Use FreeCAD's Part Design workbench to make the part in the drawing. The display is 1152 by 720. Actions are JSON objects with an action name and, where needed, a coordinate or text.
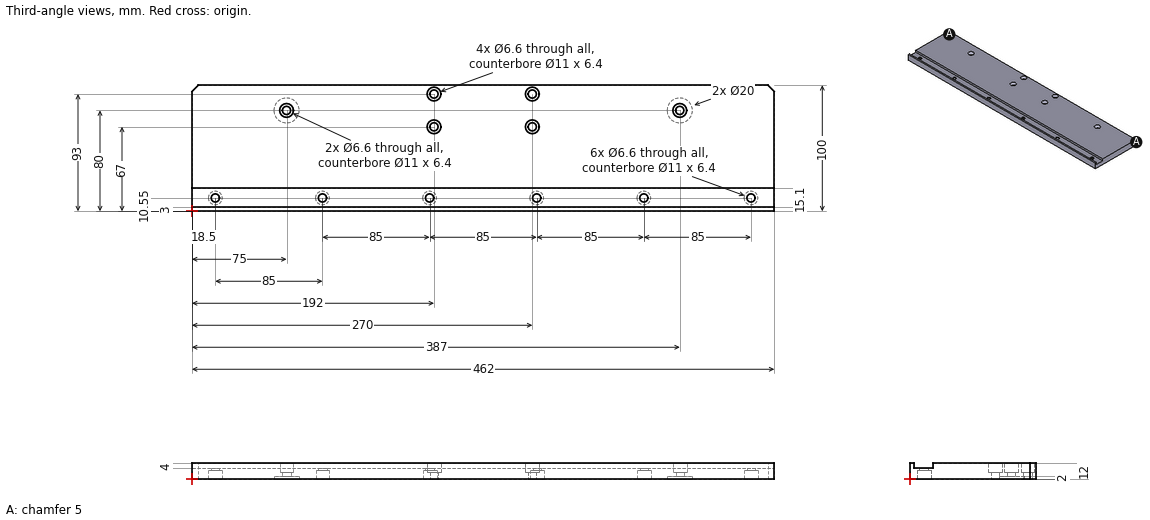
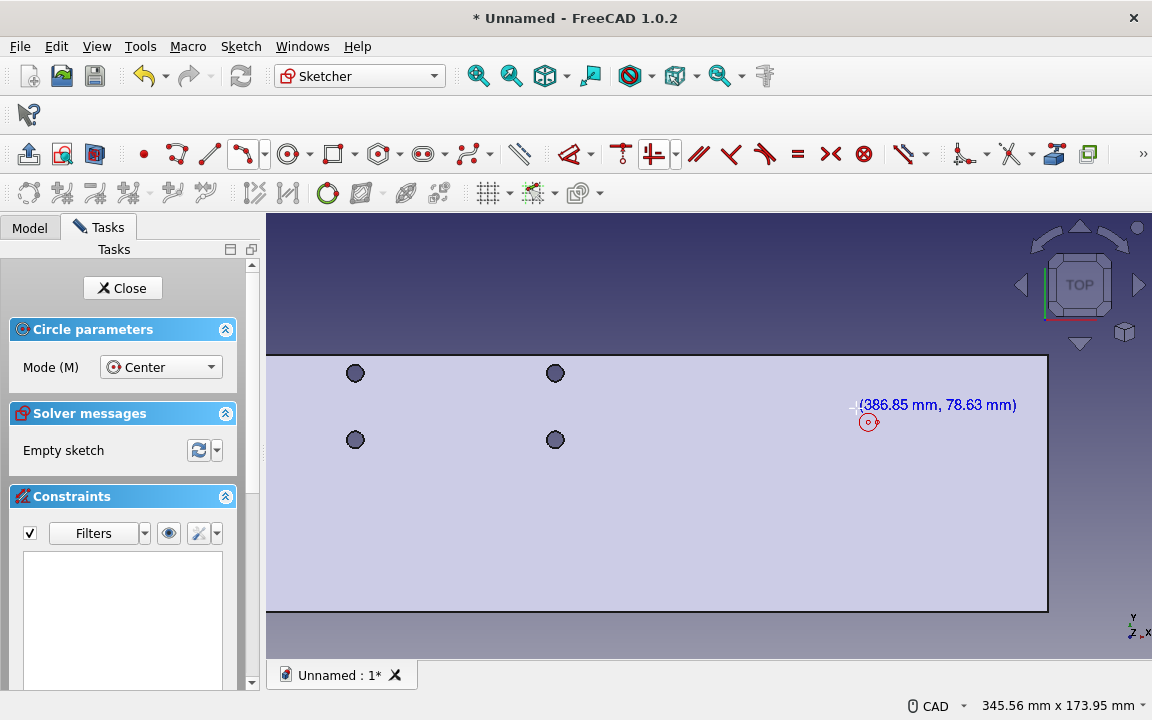
{"action": "left_click", "coordinate": [855, 406]}
{"action": "mouse_move", "coordinate": [873, 388]}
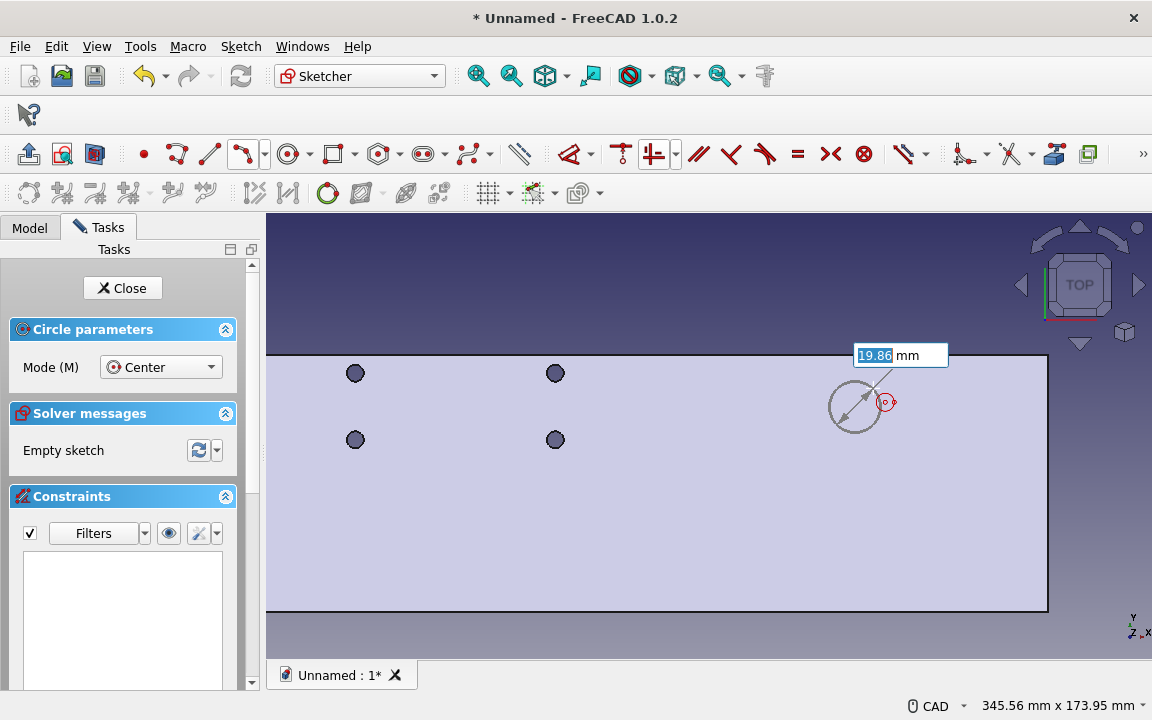
{"action": "type", "text": "20"}
{"action": "key", "text": "Return"}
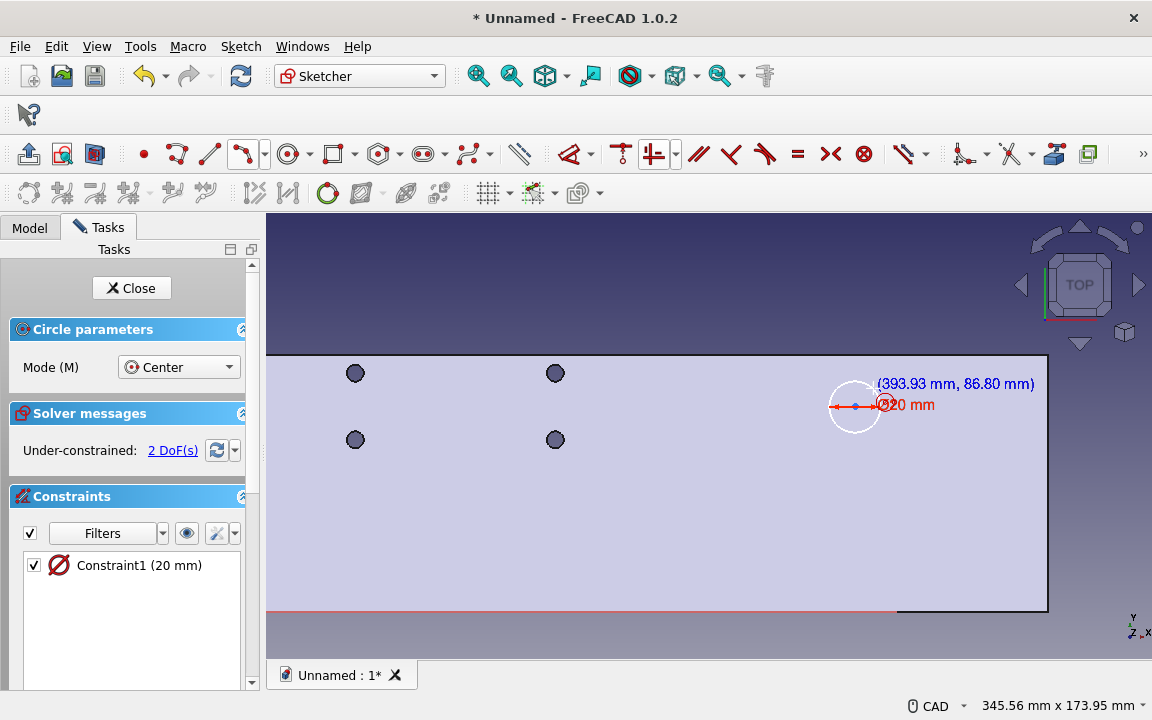
{"action": "scroll", "coordinate": [860, 387], "scroll_direction": "down", "scroll_amount": 4}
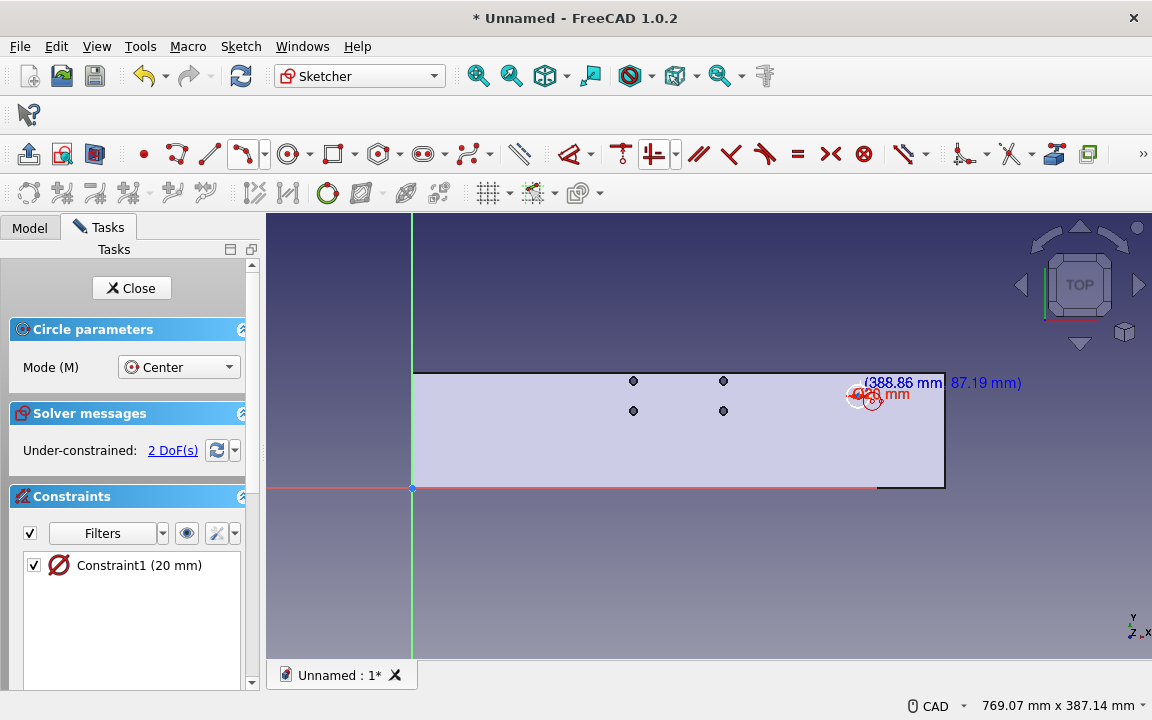
{"action": "scroll", "coordinate": [499, 396], "scroll_direction": "up", "scroll_amount": 4}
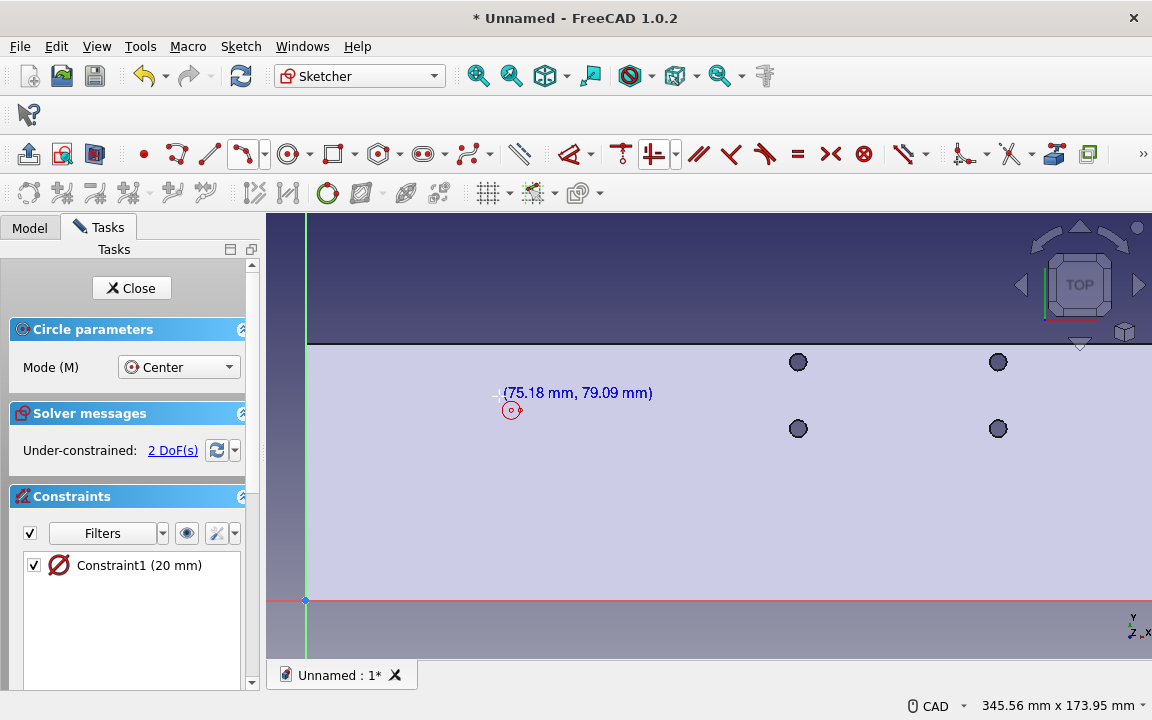
{"action": "left_click", "coordinate": [498, 395]}
{"action": "mouse_move", "coordinate": [516, 377]}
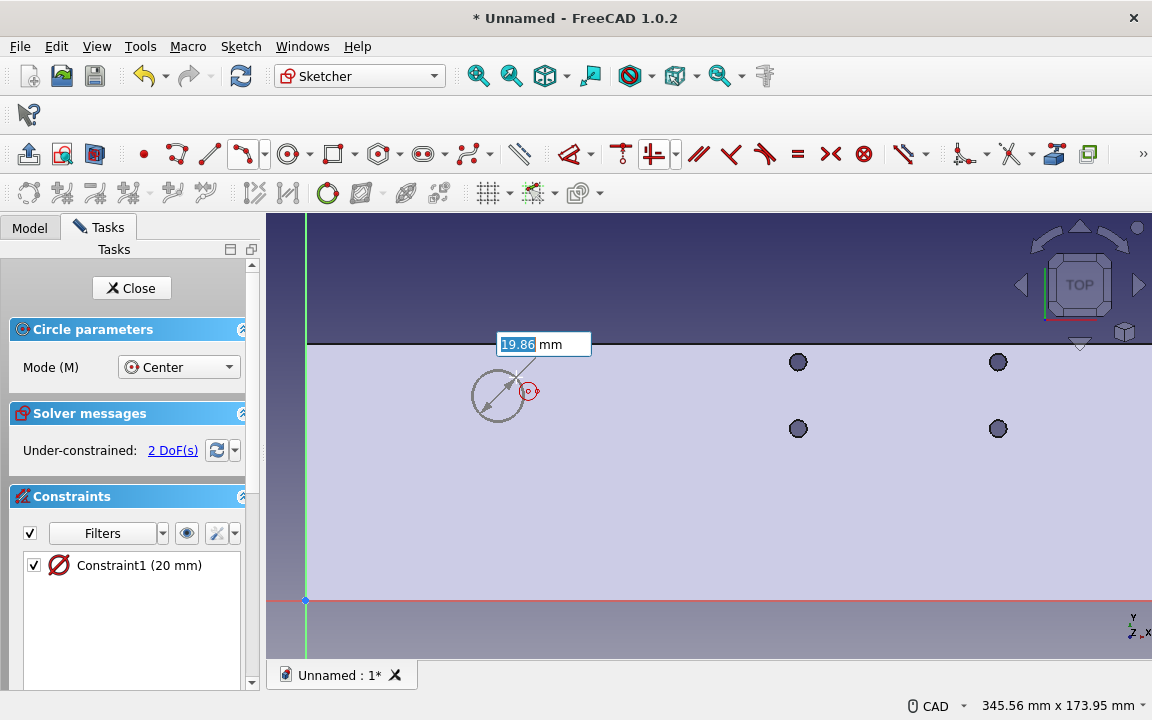
{"action": "type", "text": "20"}
{"action": "key", "text": "Return"}
{"action": "key", "text": "Escape"}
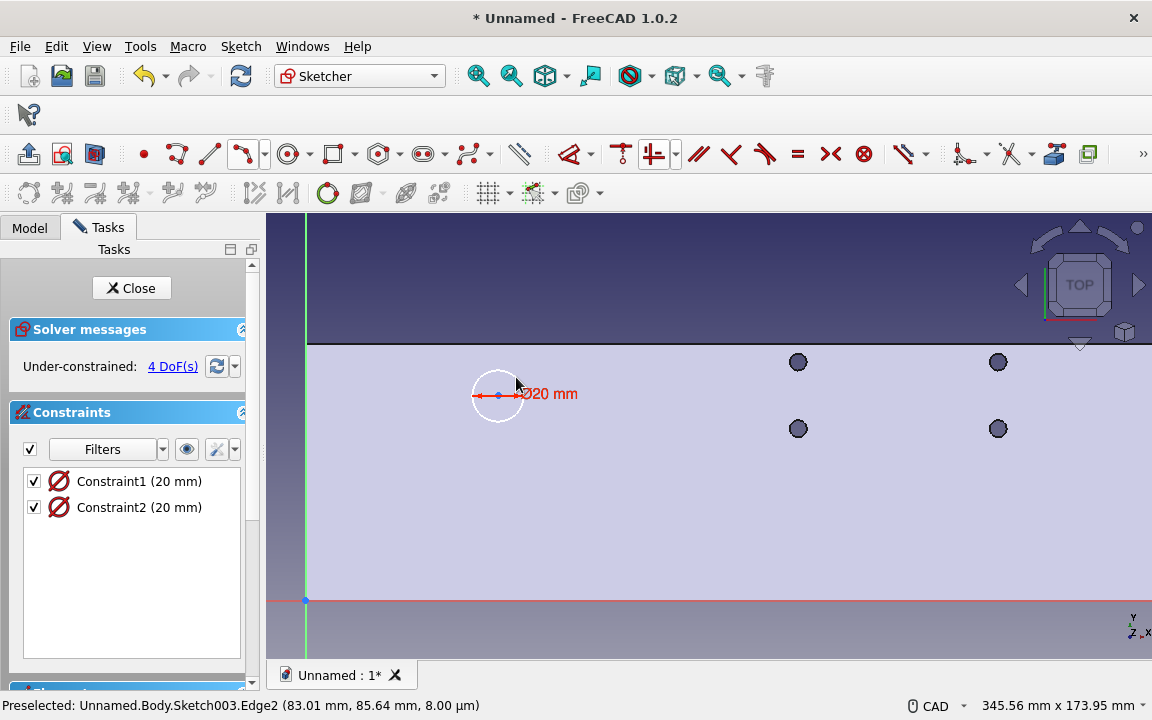
{"action": "scroll", "coordinate": [498, 396], "scroll_direction": "down", "scroll_amount": 4}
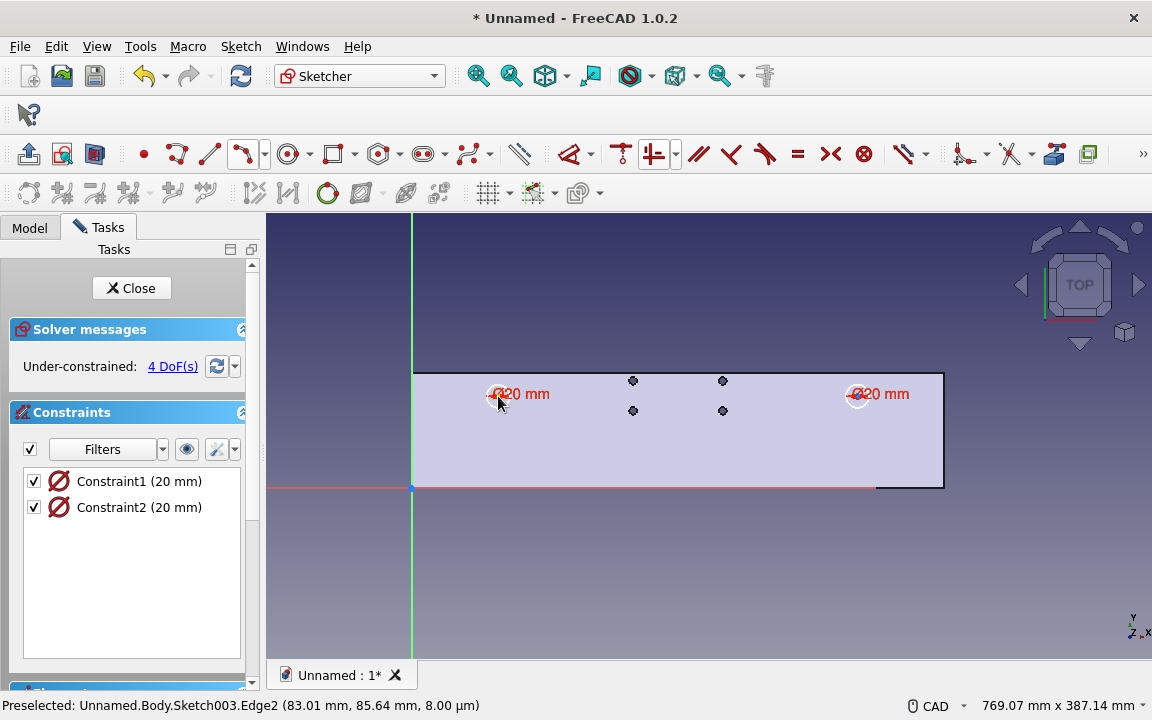
{"action": "left_click", "coordinate": [858, 396]}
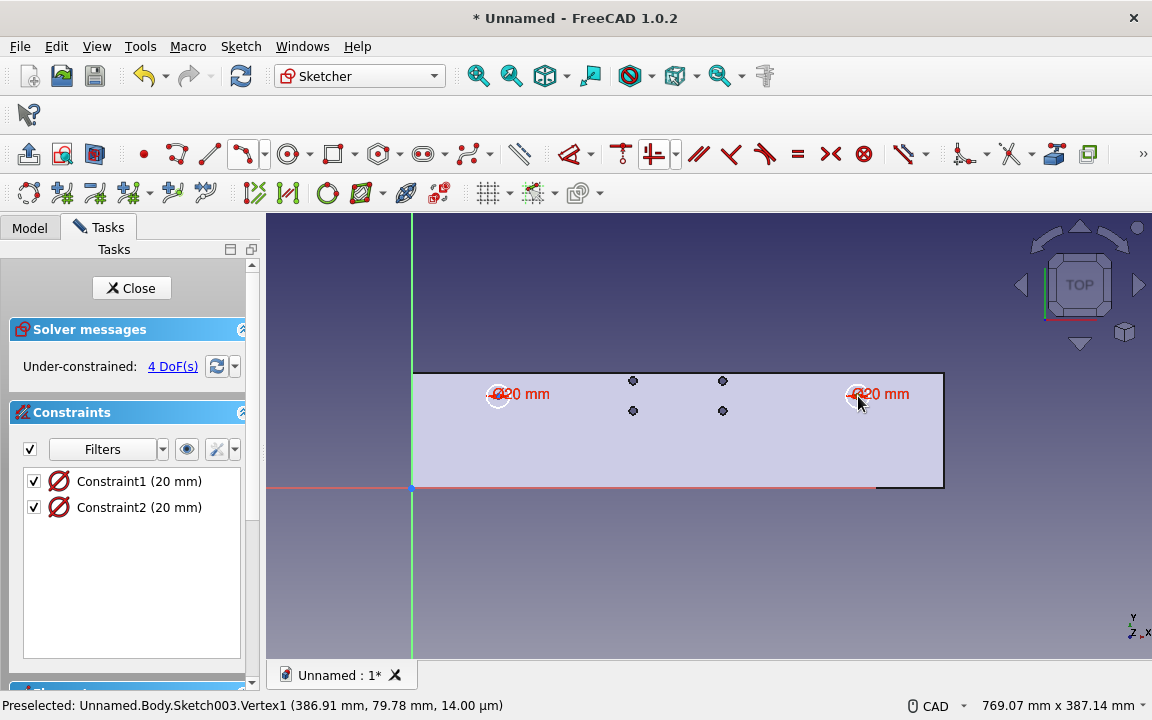
{"action": "left_click", "coordinate": [498, 396]}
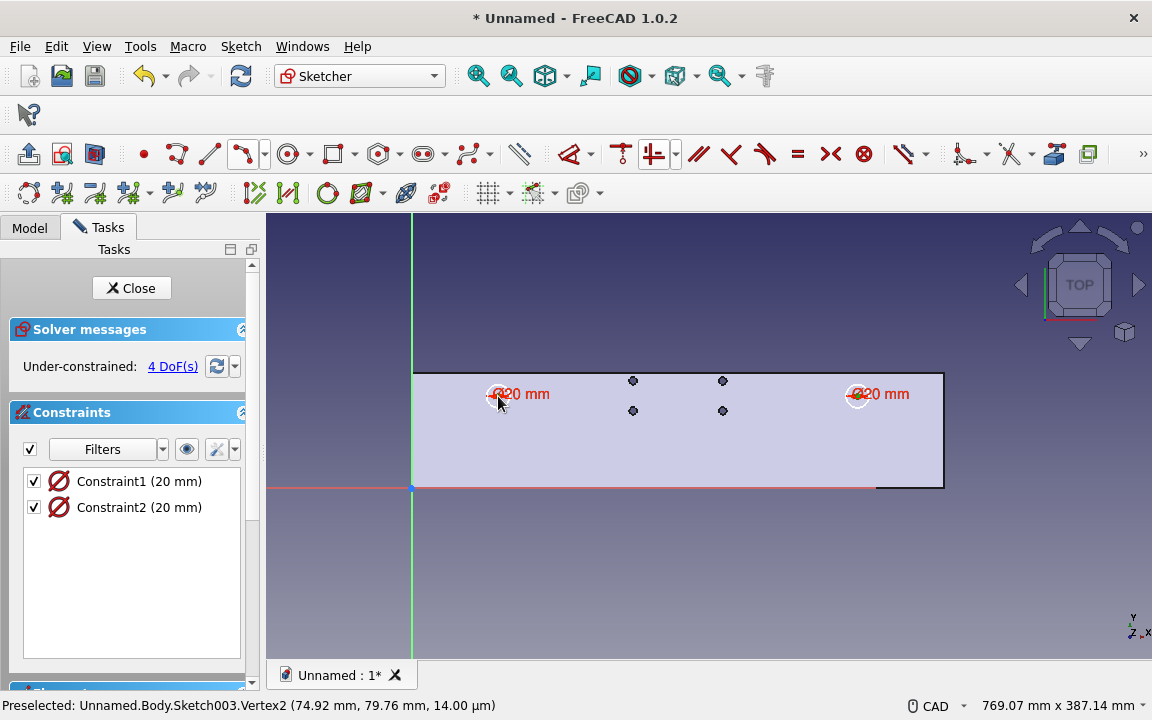
{"action": "left_click", "coordinate": [676, 154]}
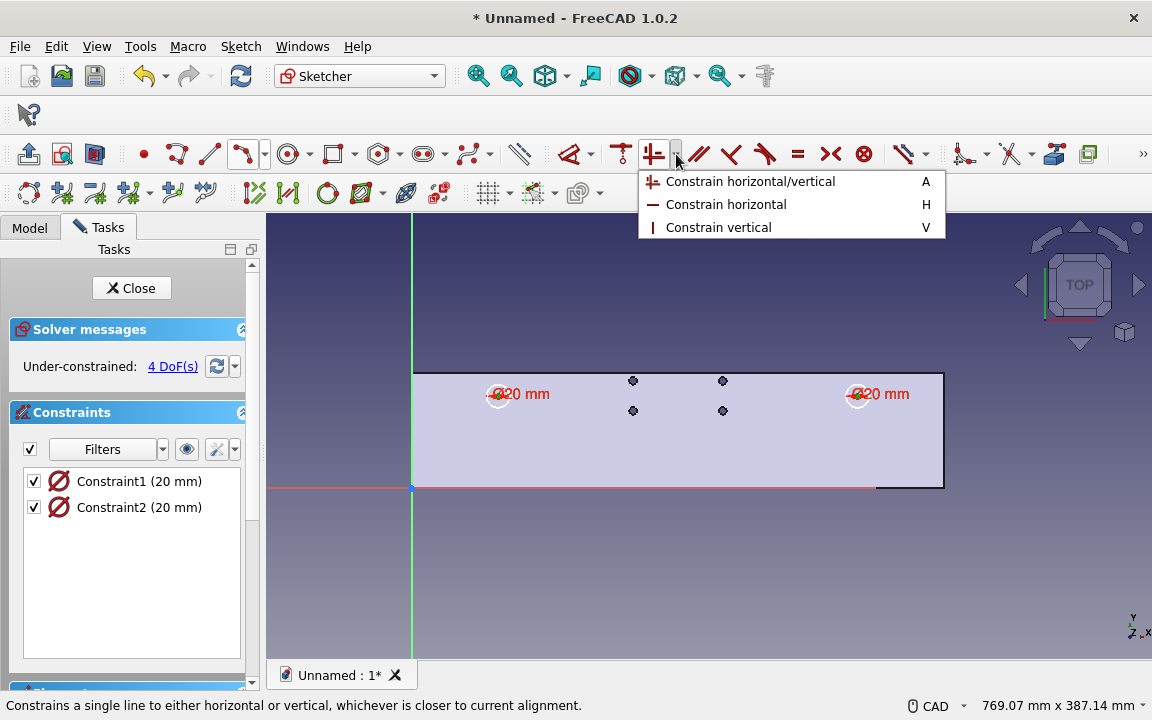
{"action": "left_click", "coordinate": [792, 204]}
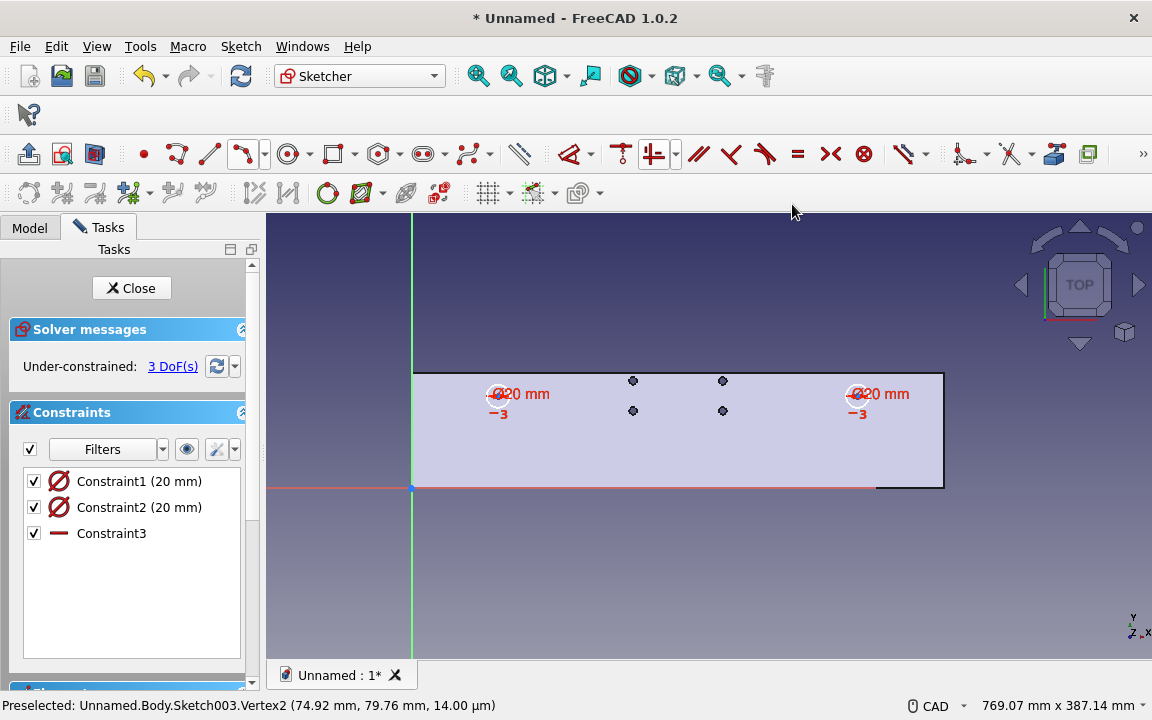
{"action": "left_click", "coordinate": [568, 154]}